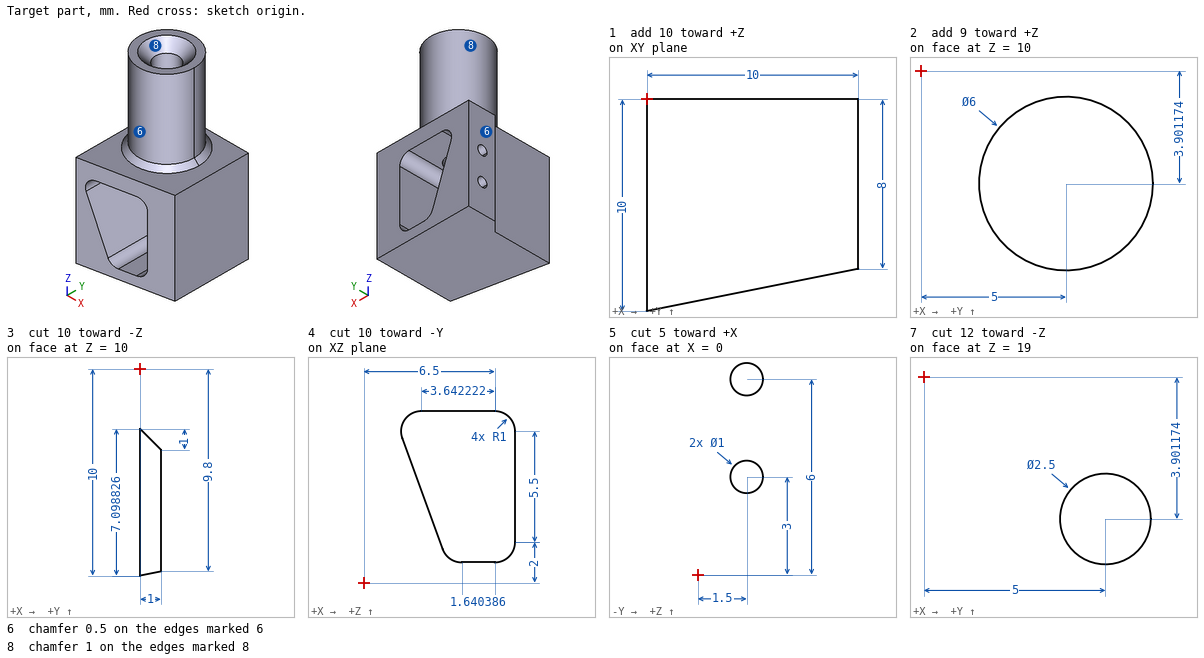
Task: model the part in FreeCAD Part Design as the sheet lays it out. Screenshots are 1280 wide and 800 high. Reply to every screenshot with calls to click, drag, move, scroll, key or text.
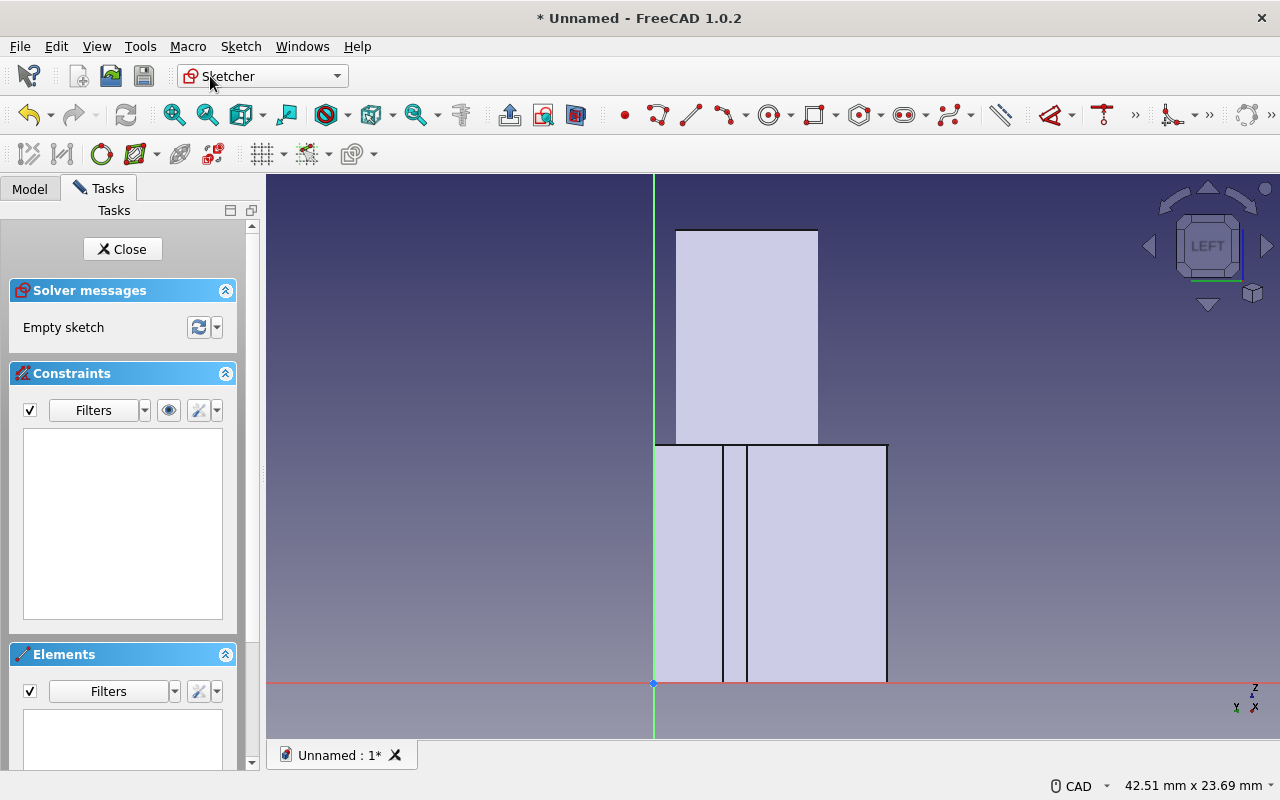
scroll(656, 711, up, 4)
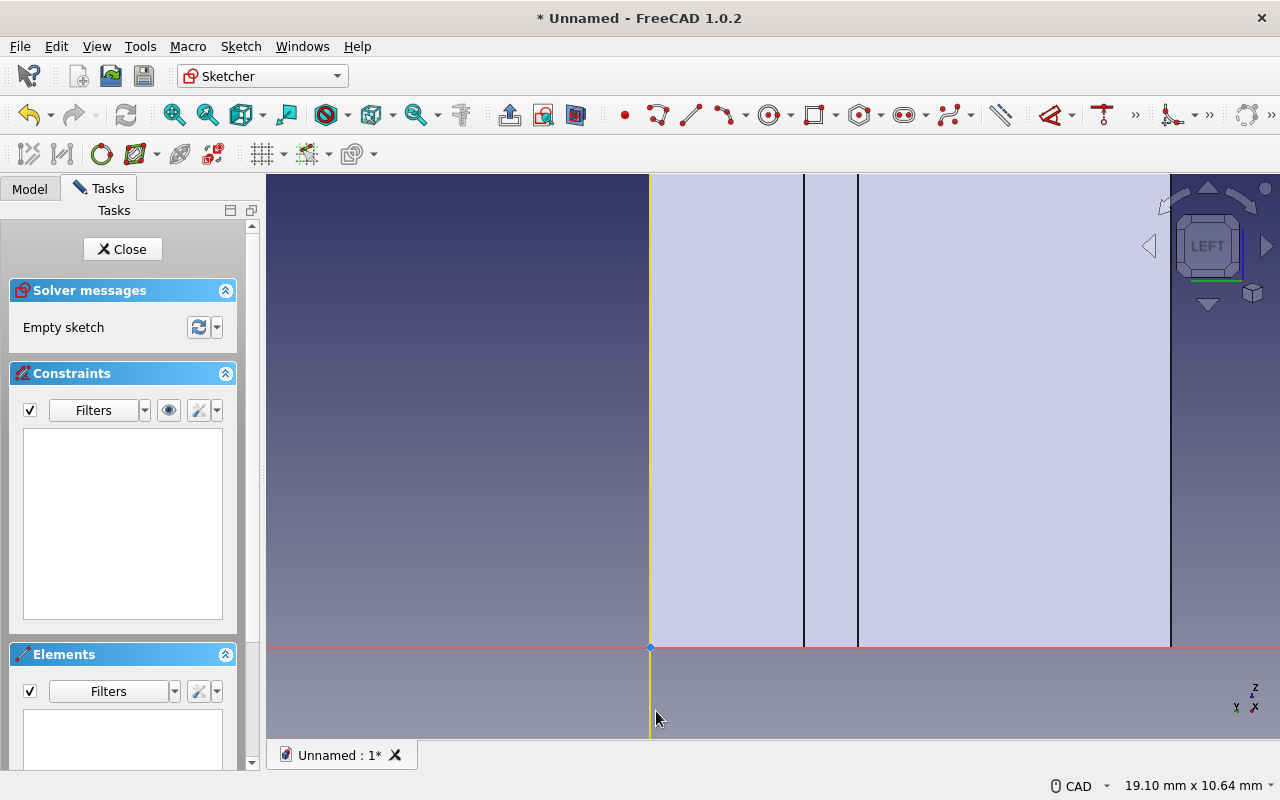
key(g)
key(c)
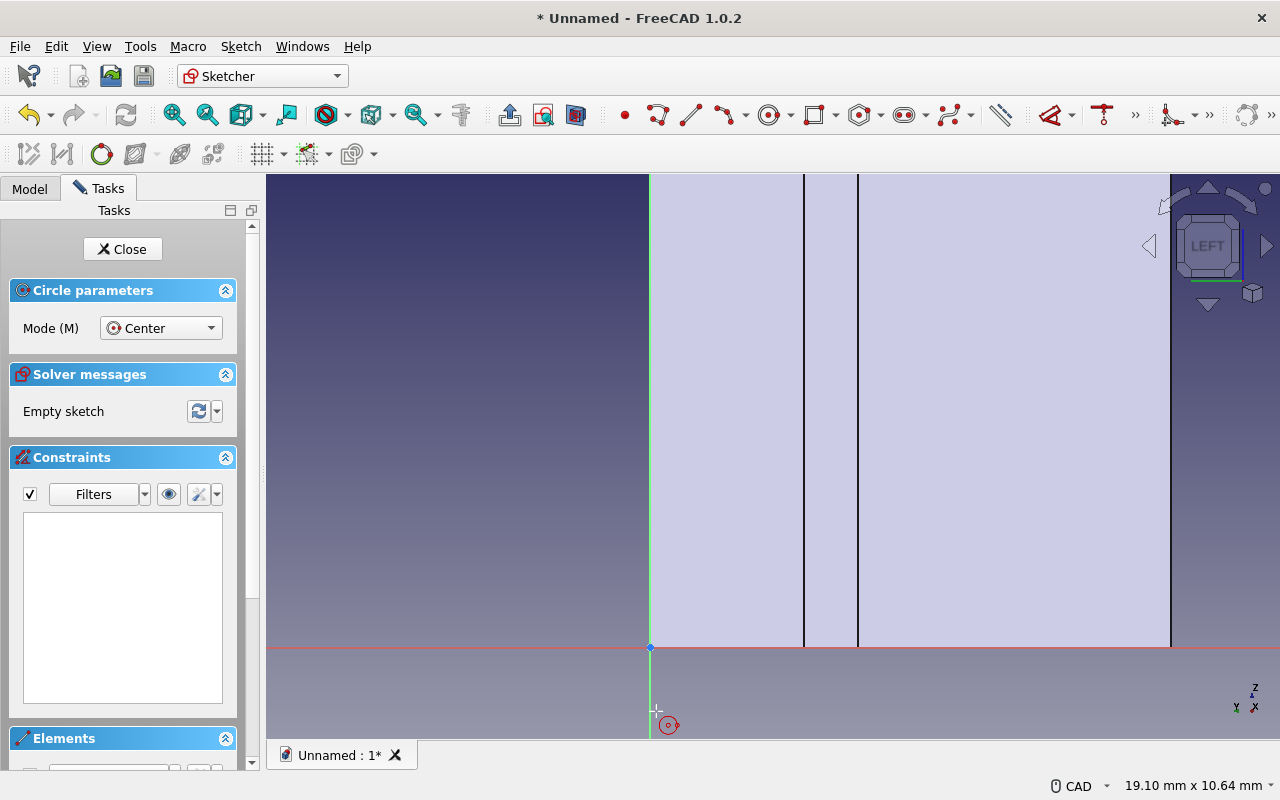
click(730, 489)
click(749, 470)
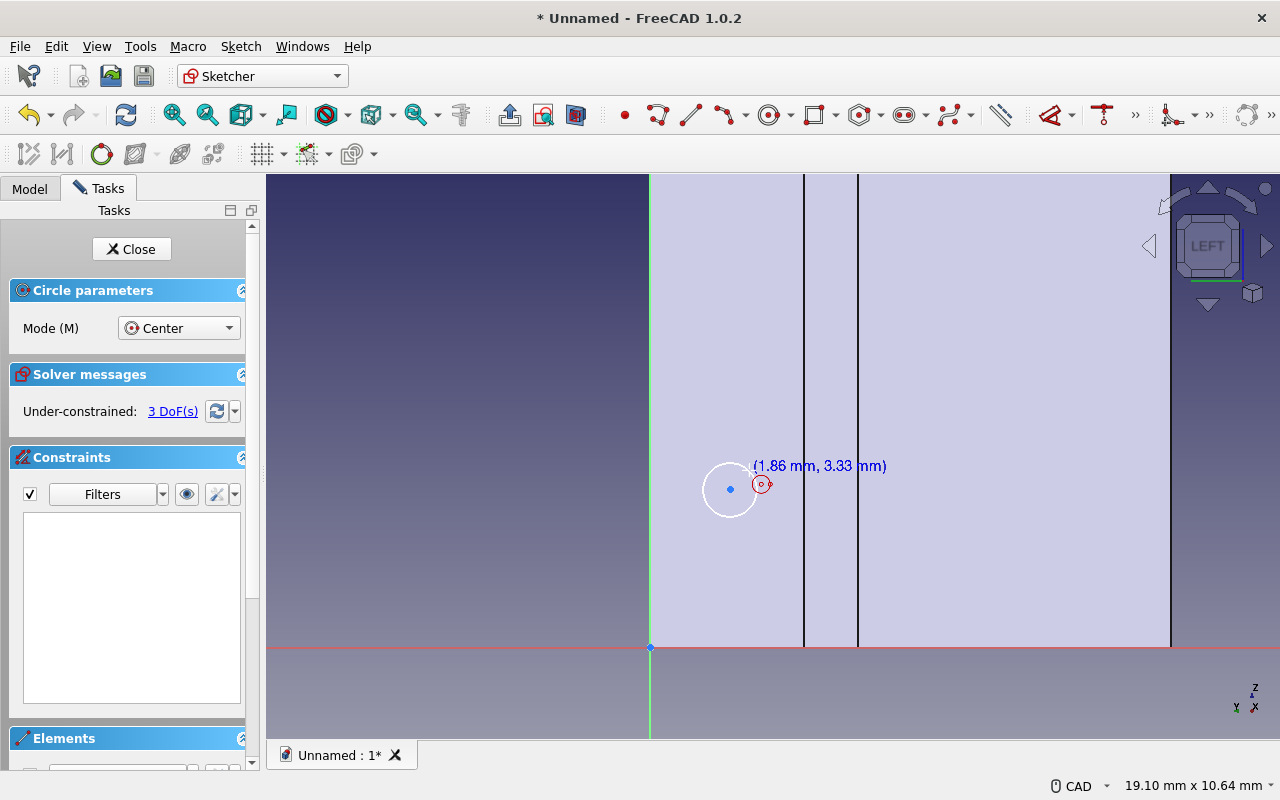
click(730, 329)
click(749, 310)
key(Escape)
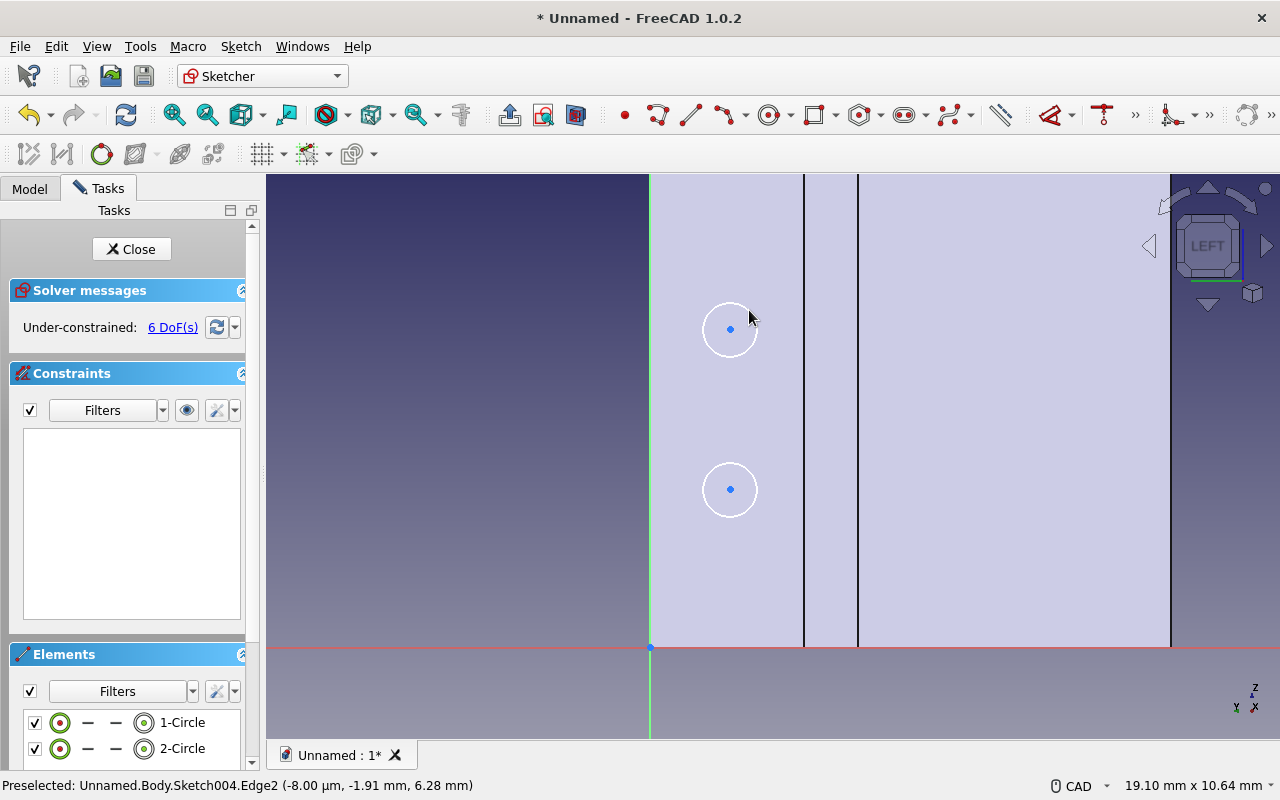
click(749, 471)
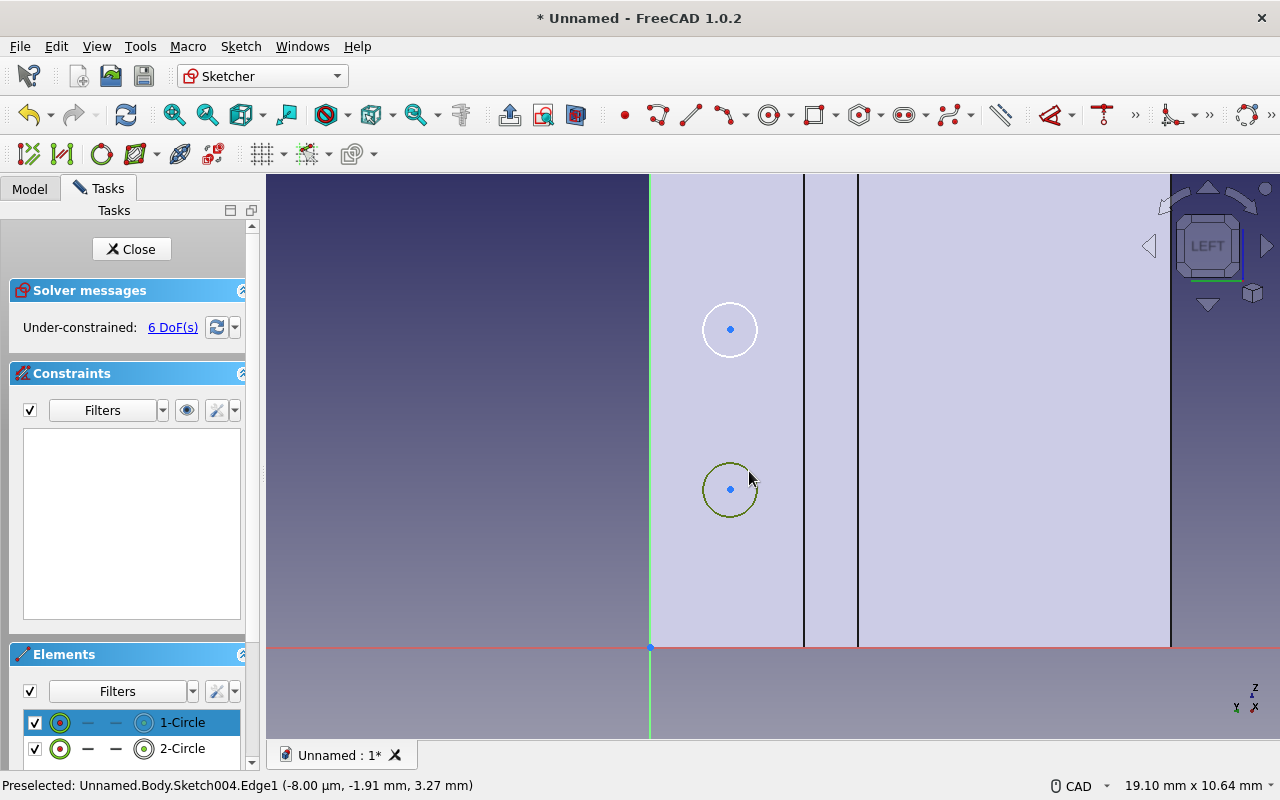
click(749, 311)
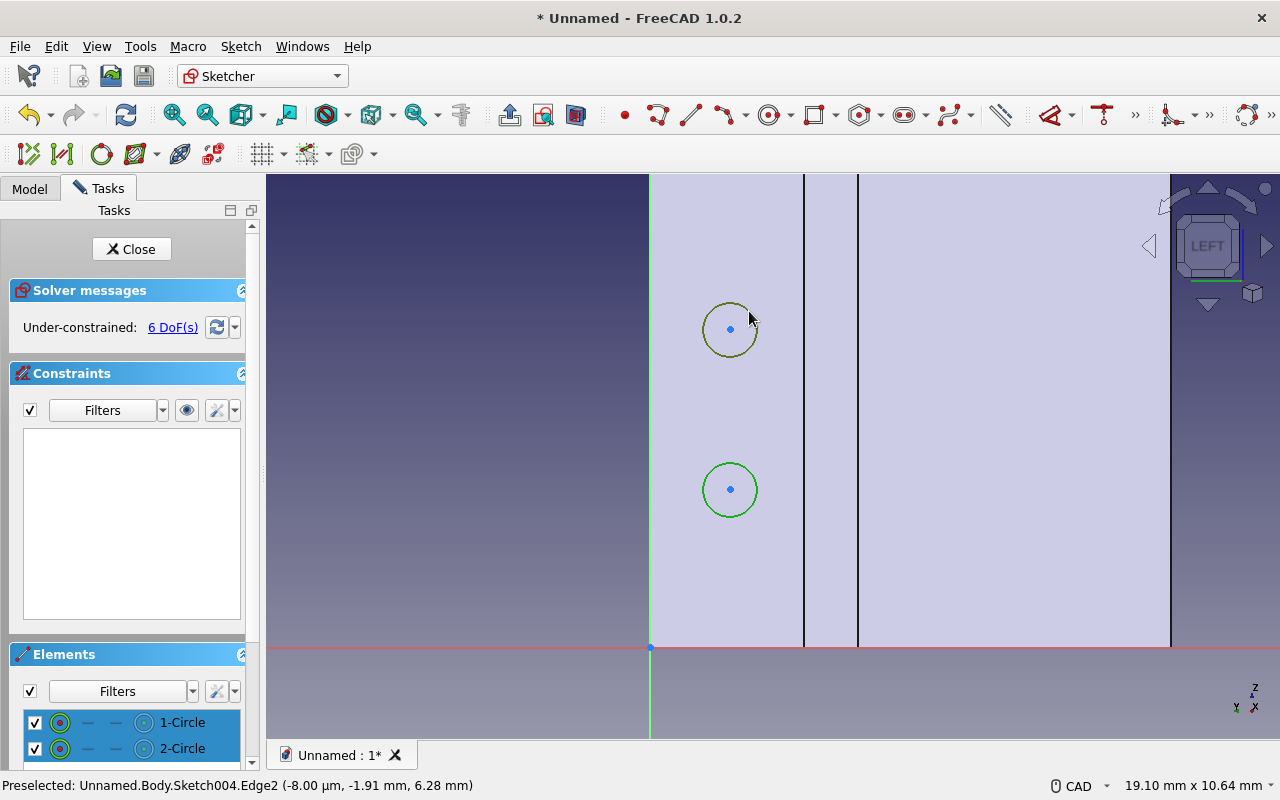
key(e)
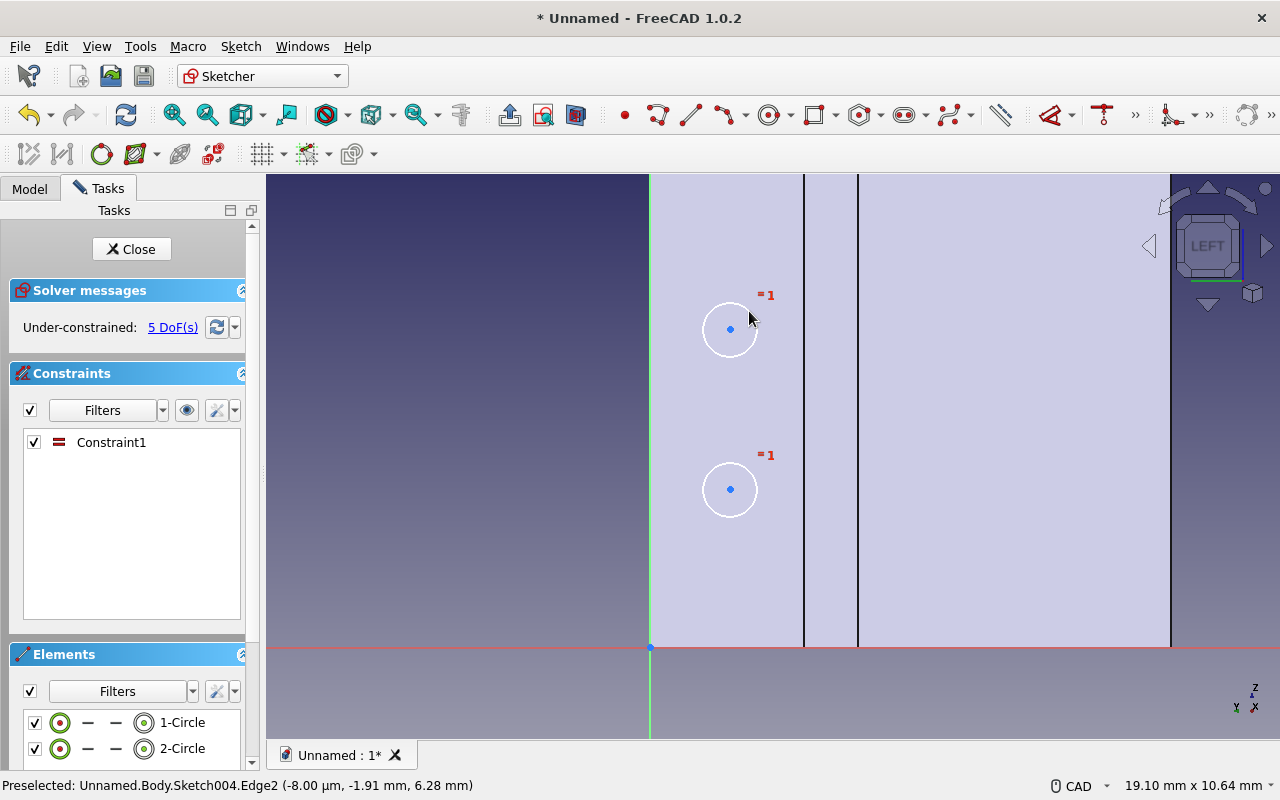
click(730, 490)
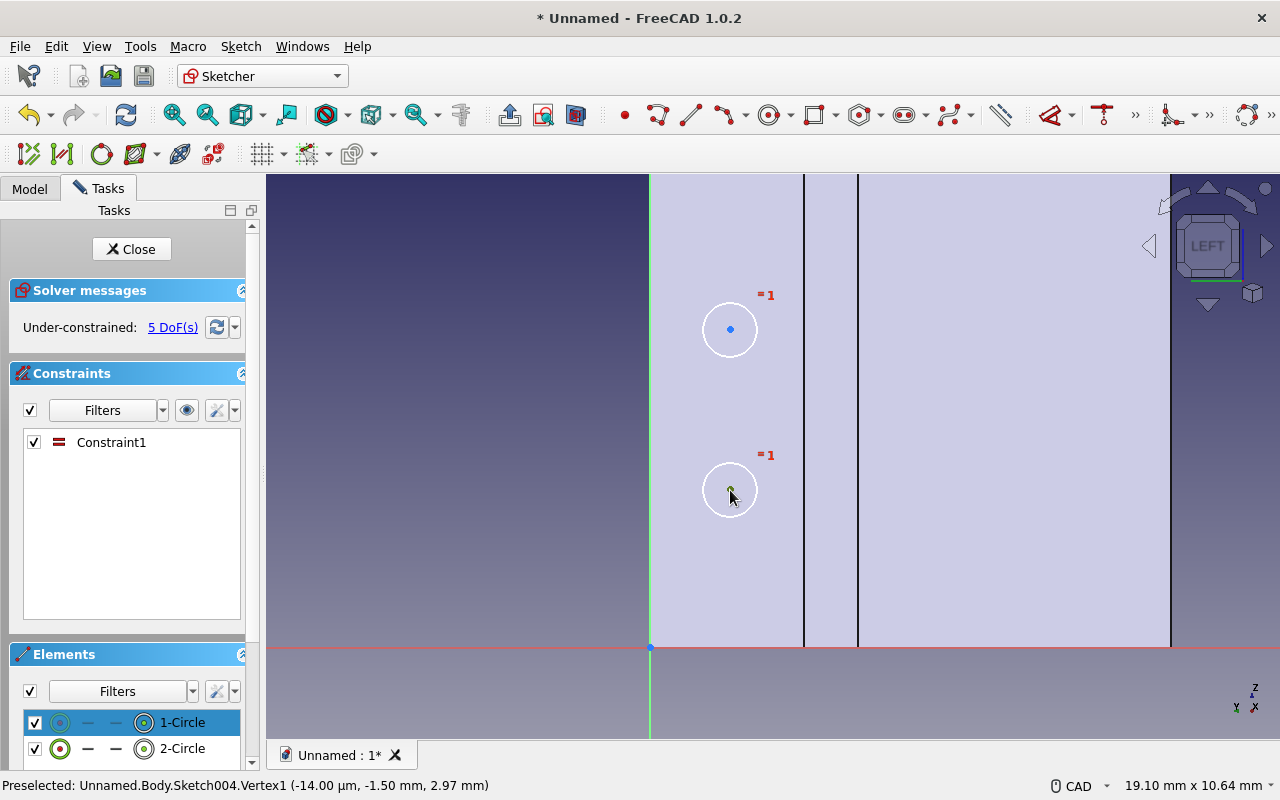
click(730, 330)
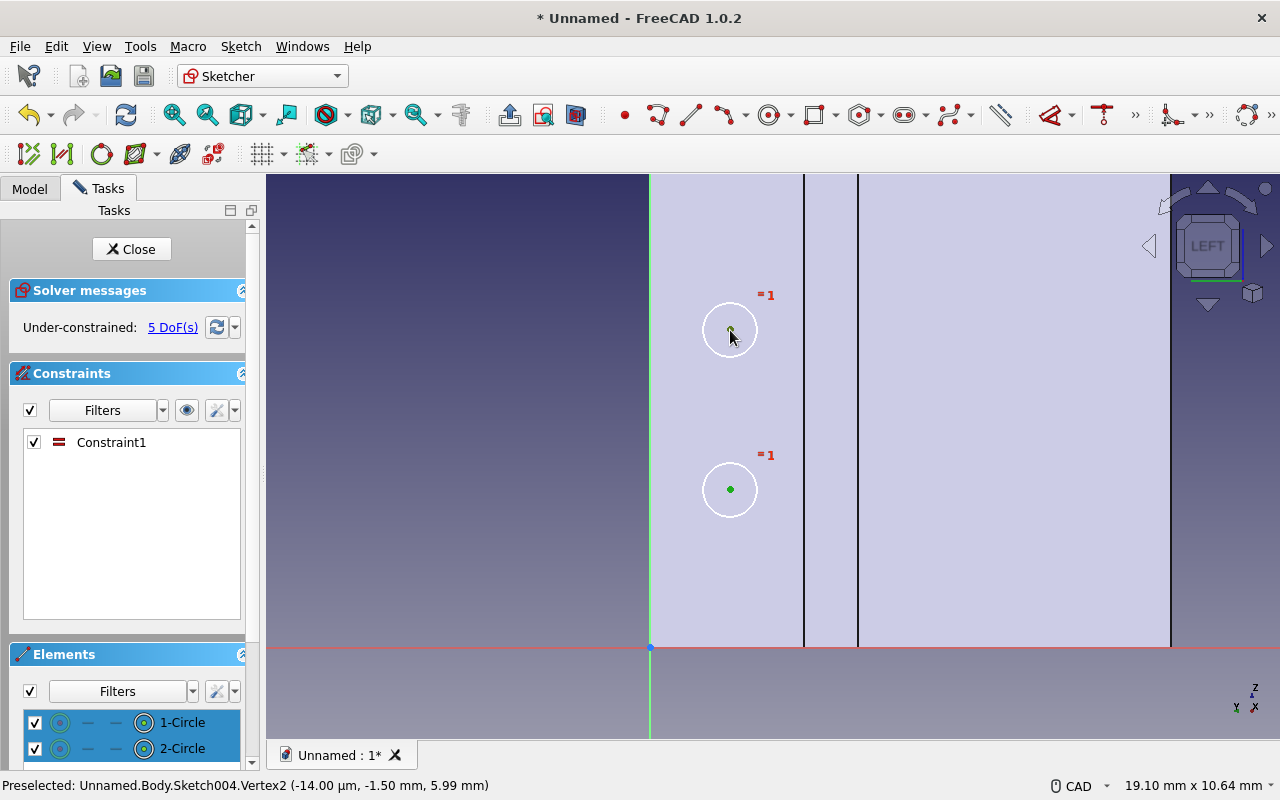
key(v)